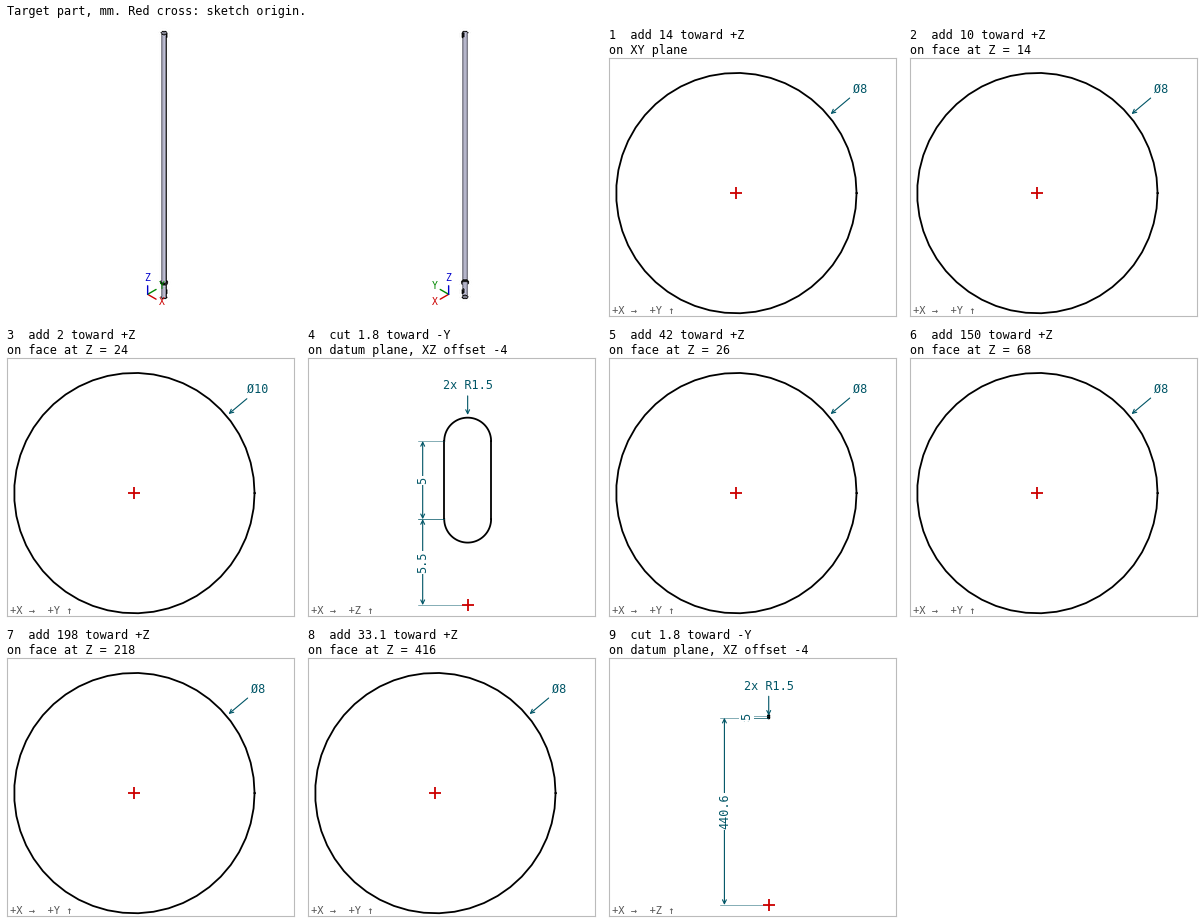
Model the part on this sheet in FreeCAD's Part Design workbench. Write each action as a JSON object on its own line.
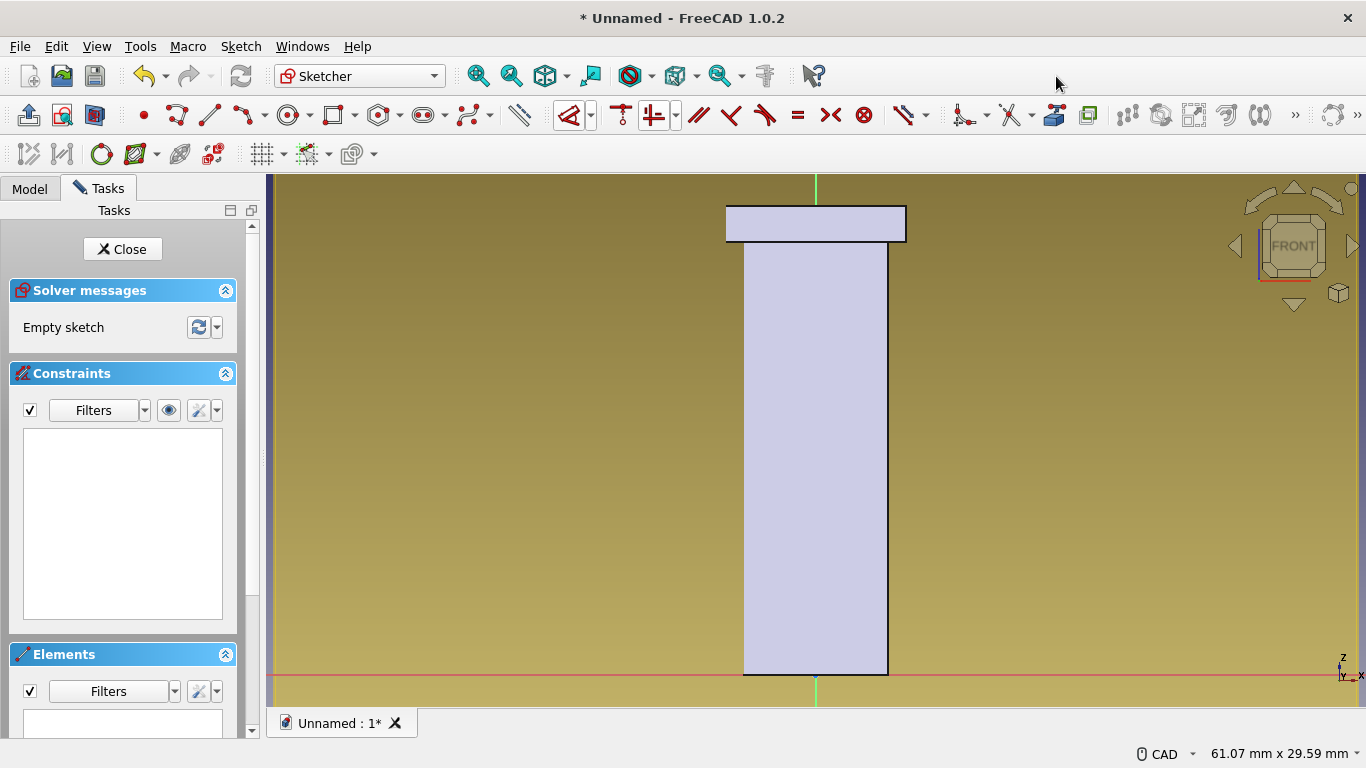
{"action": "left_click", "coordinate": [95, 116]}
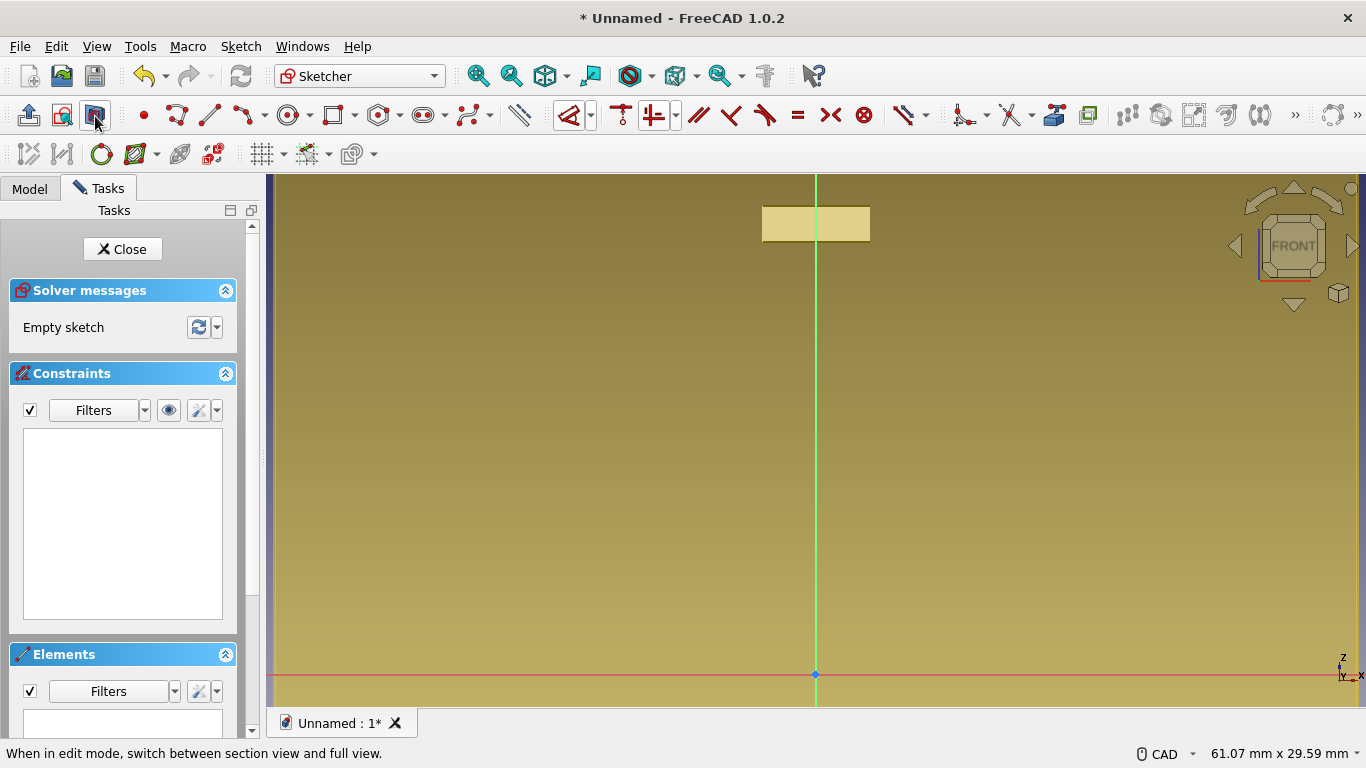
{"action": "scroll", "coordinate": [439, 202], "scroll_direction": "down", "scroll_amount": 1}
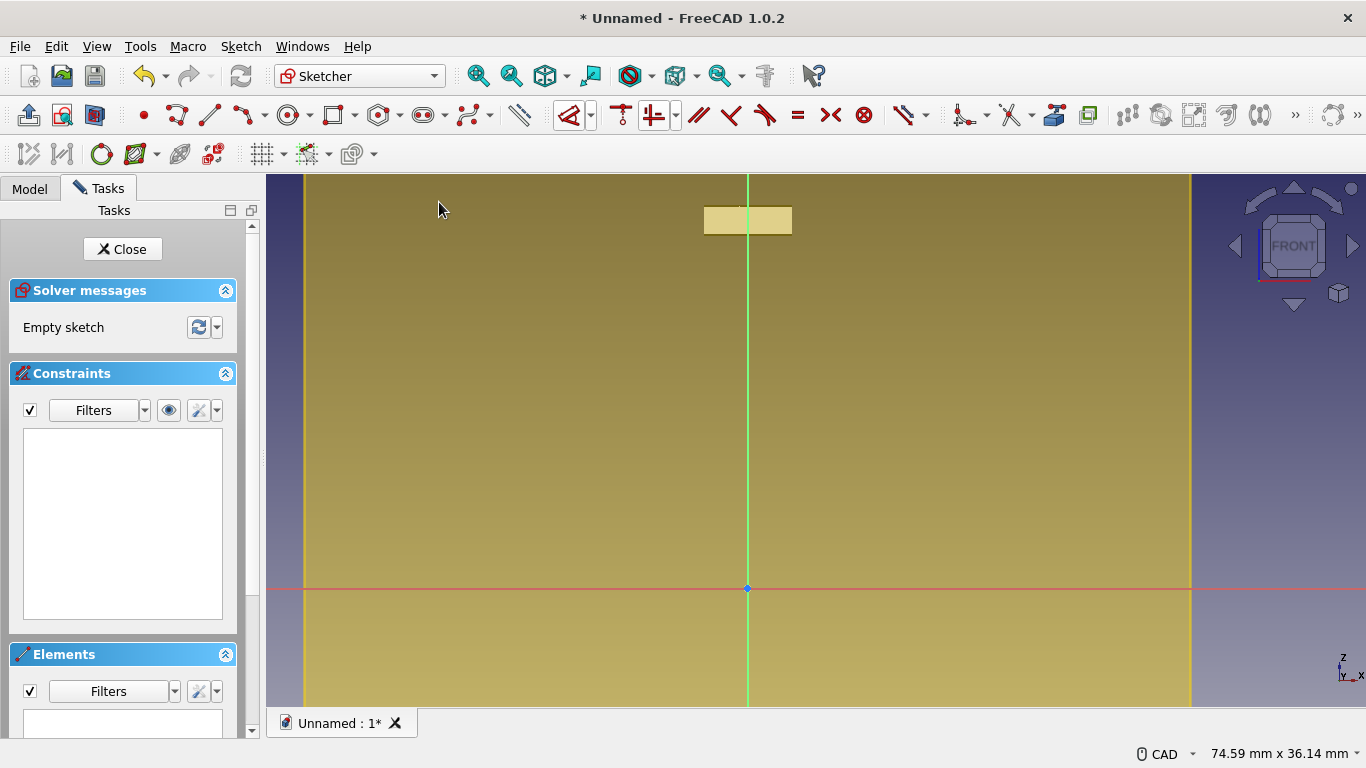
{"action": "scroll", "coordinate": [748, 574], "scroll_direction": "up", "scroll_amount": 3}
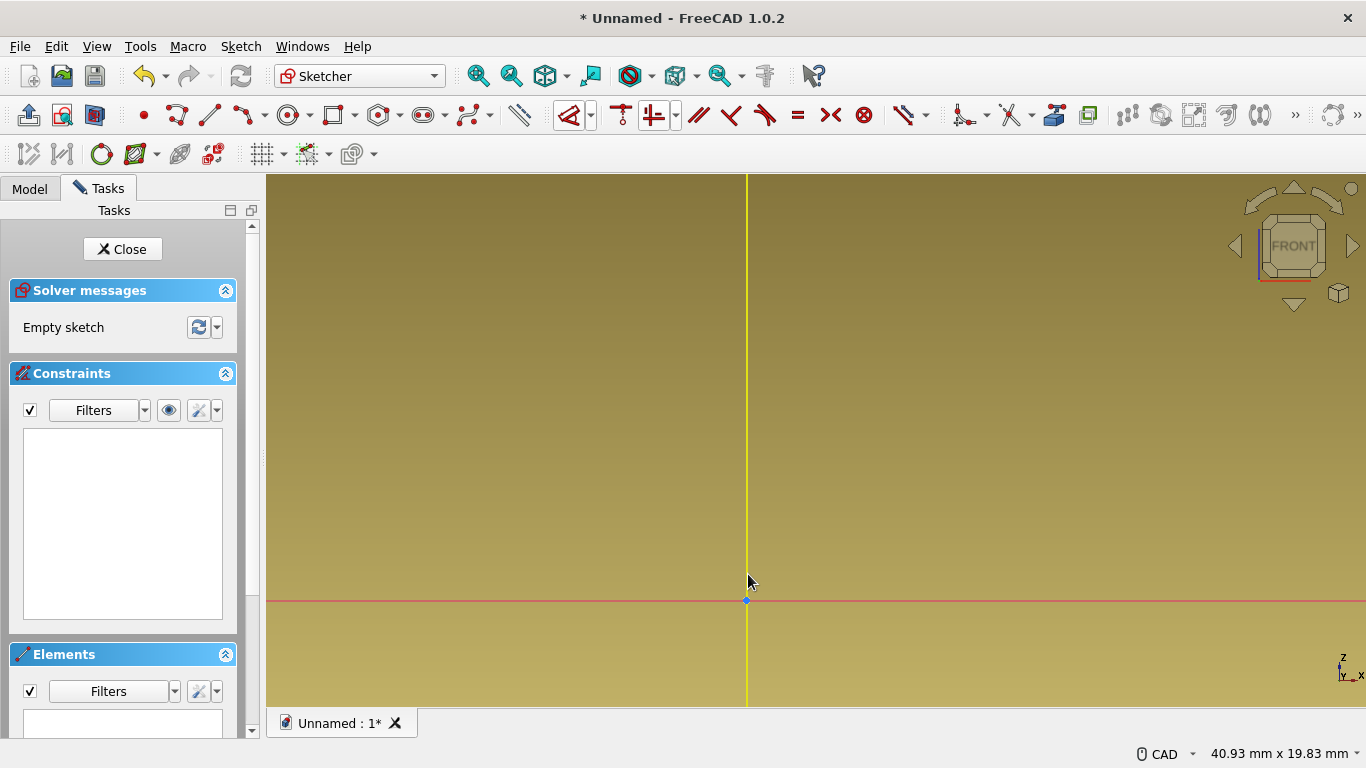
{"action": "left_click", "coordinate": [422, 116]}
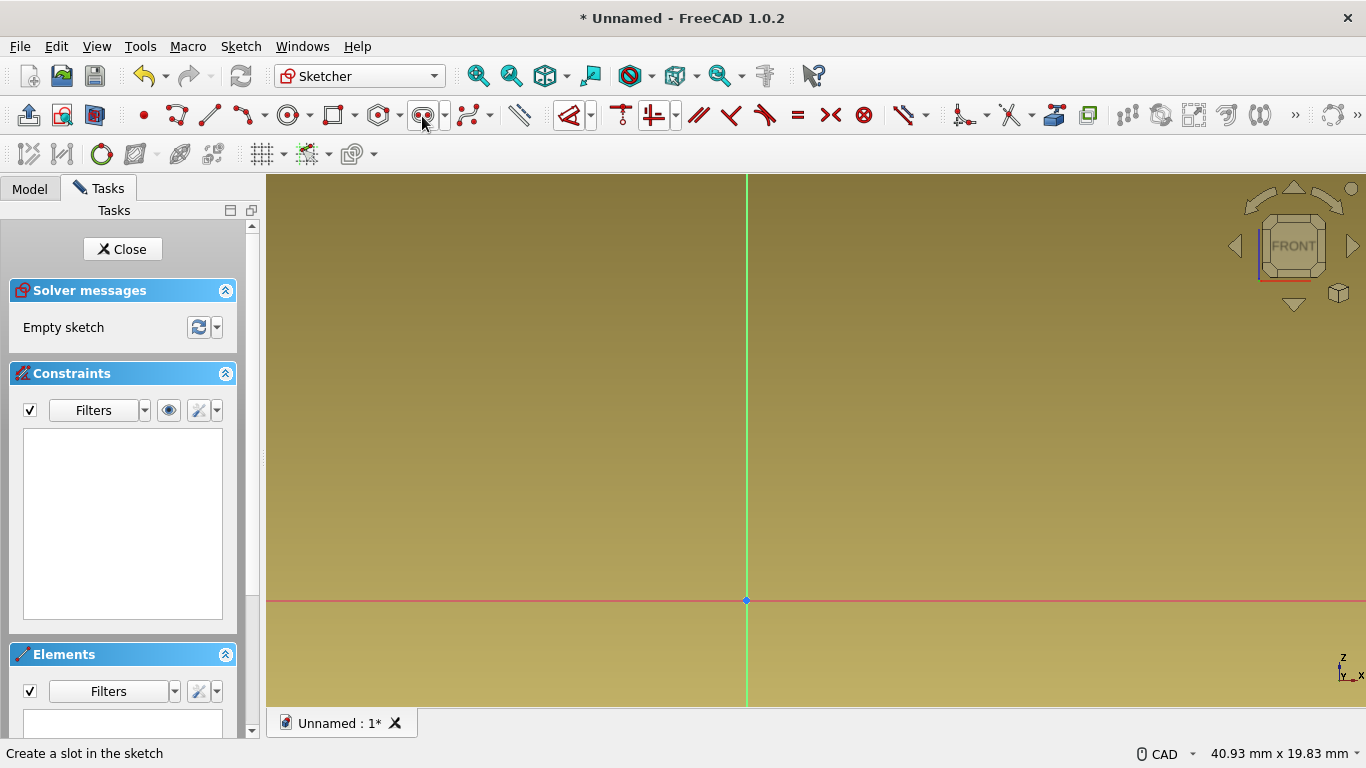
{"action": "left_click", "coordinate": [747, 453]}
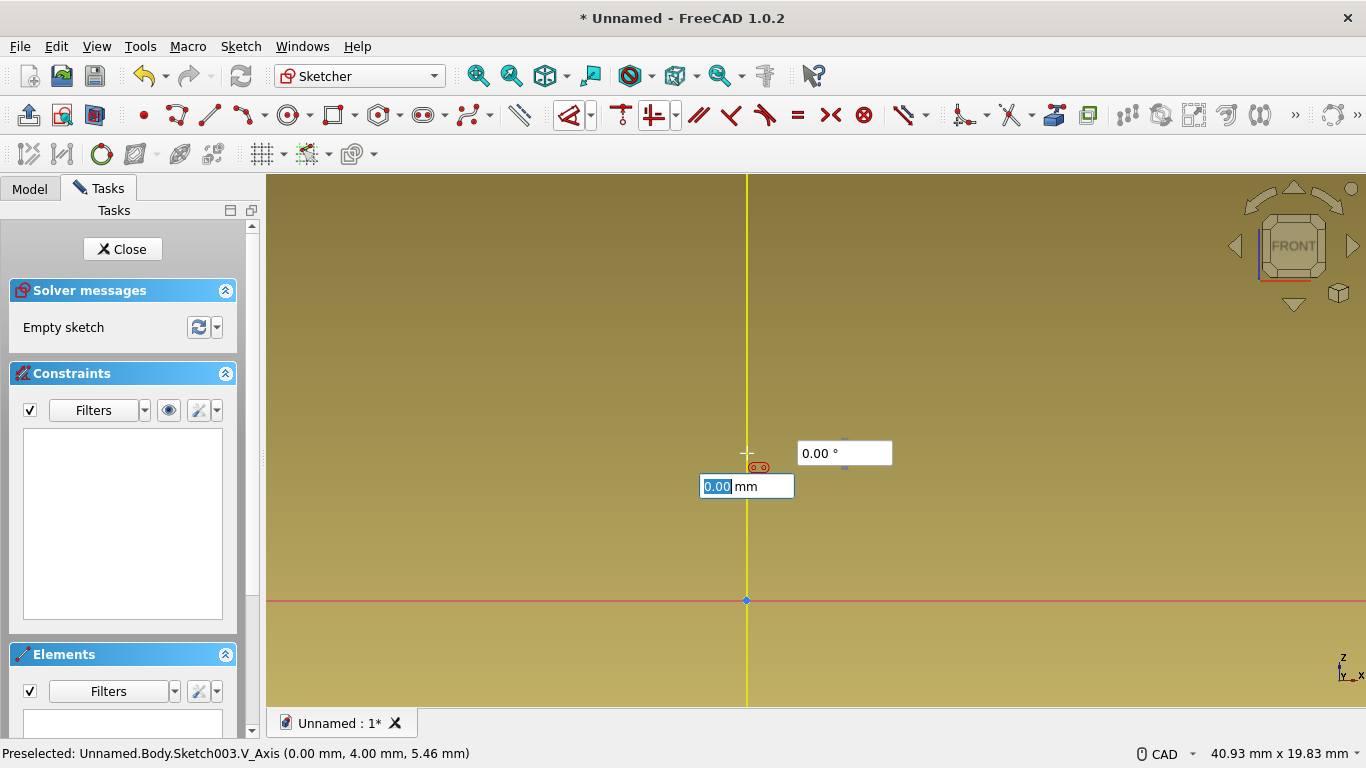
{"action": "left_click", "coordinate": [756, 319]}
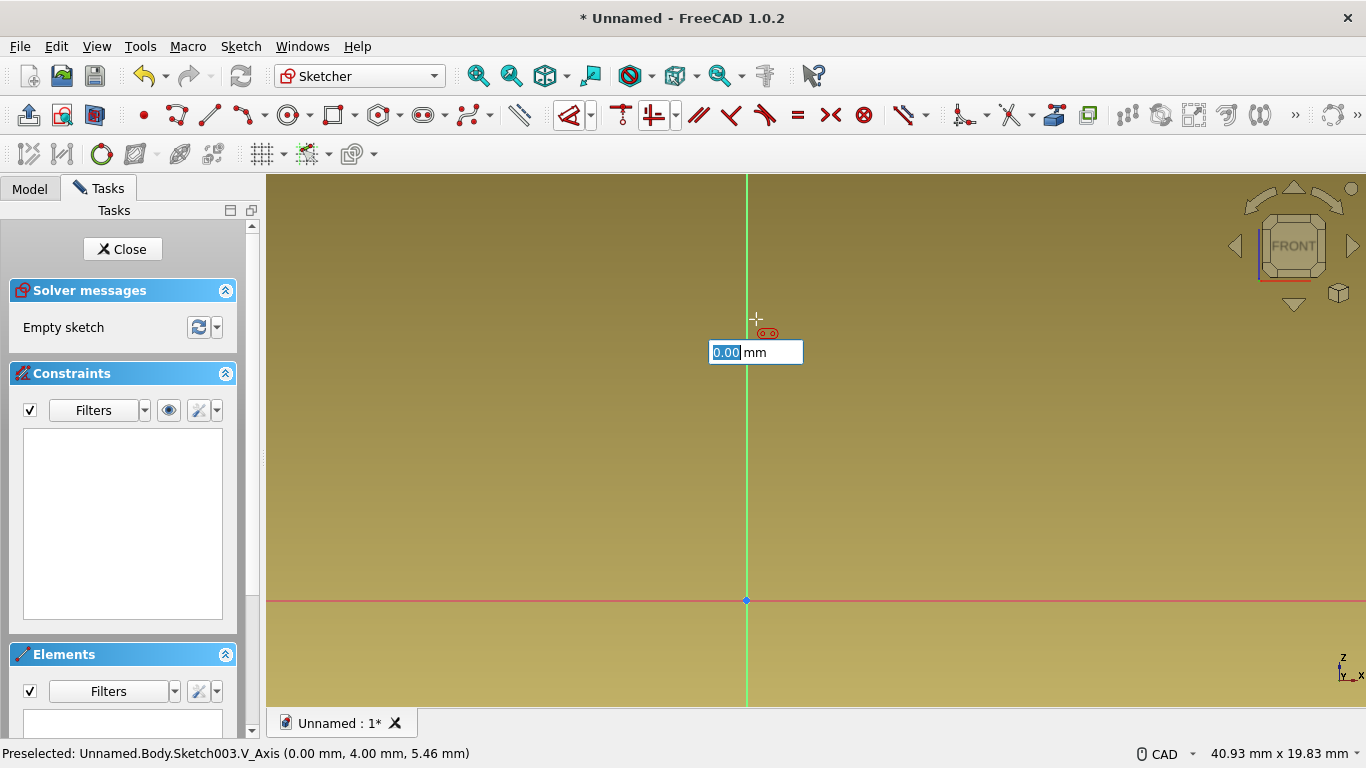
{"action": "left_click", "coordinate": [787, 386]}
{"action": "key", "text": "Escape"}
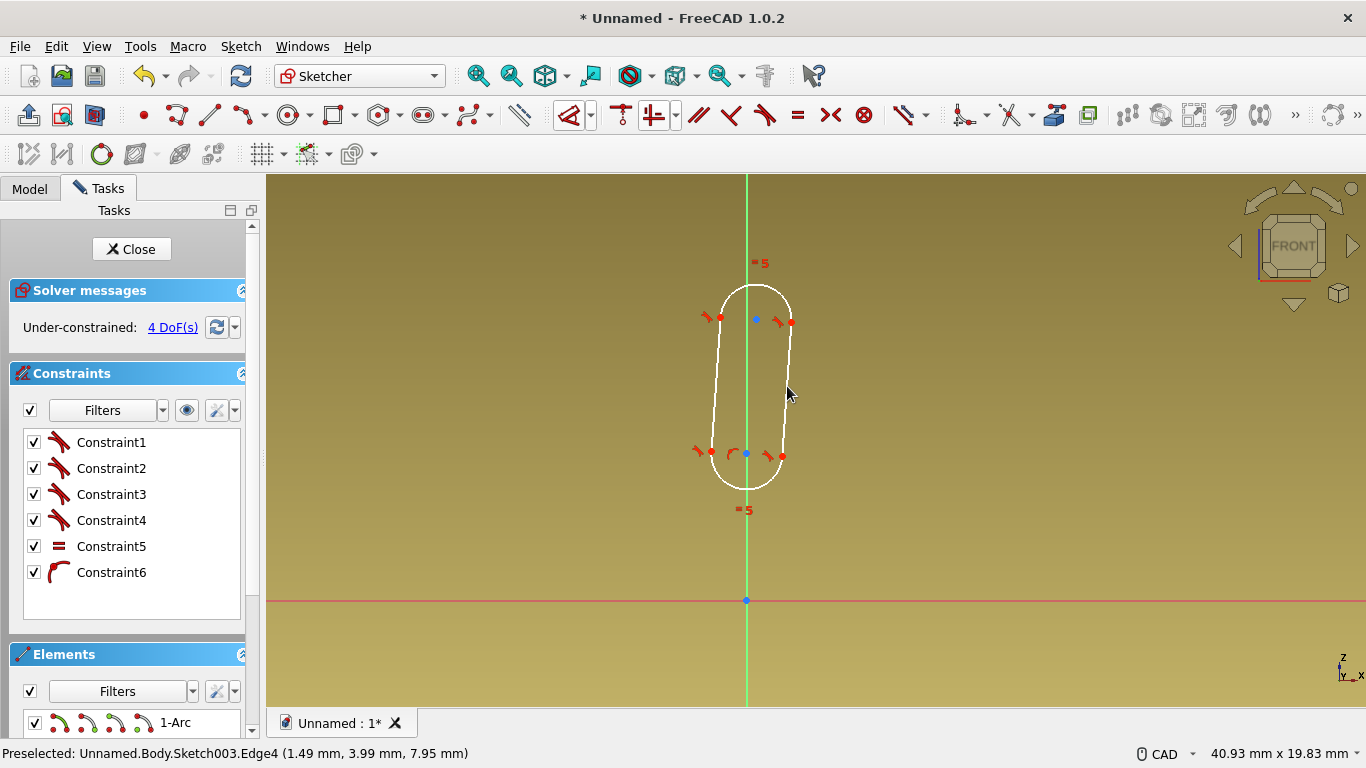
{"action": "left_click", "coordinate": [714, 411]}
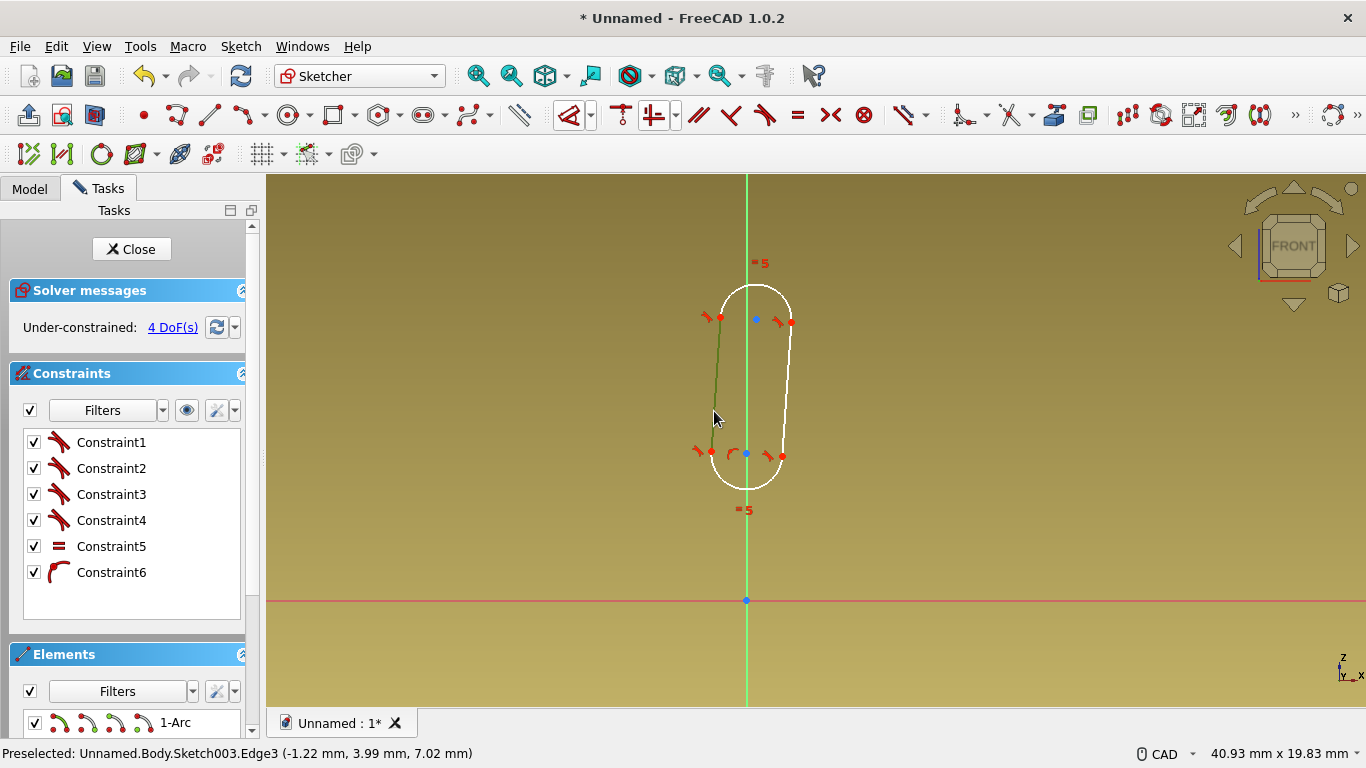
{"action": "left_click", "coordinate": [676, 116]}